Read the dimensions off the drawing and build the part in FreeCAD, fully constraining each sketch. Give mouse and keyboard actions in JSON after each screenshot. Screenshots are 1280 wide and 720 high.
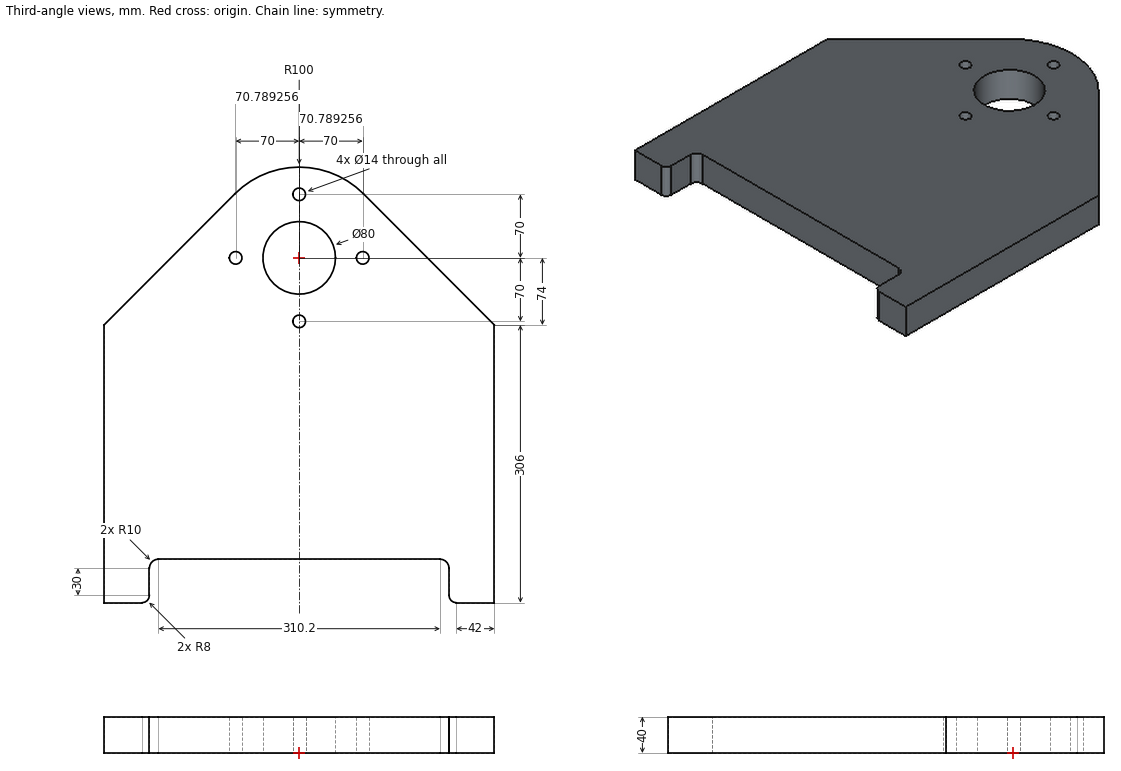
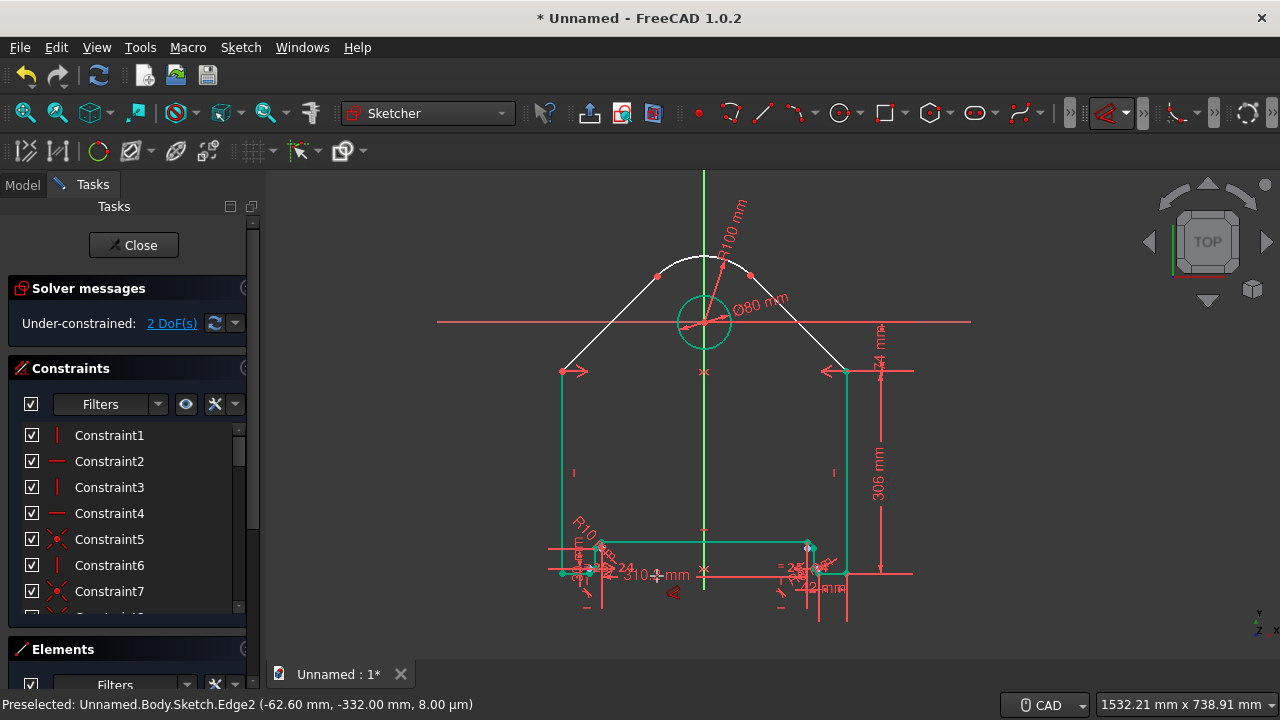
{"action": "left_click", "coordinate": [751, 275]}
{"action": "left_click", "coordinate": [728, 356]}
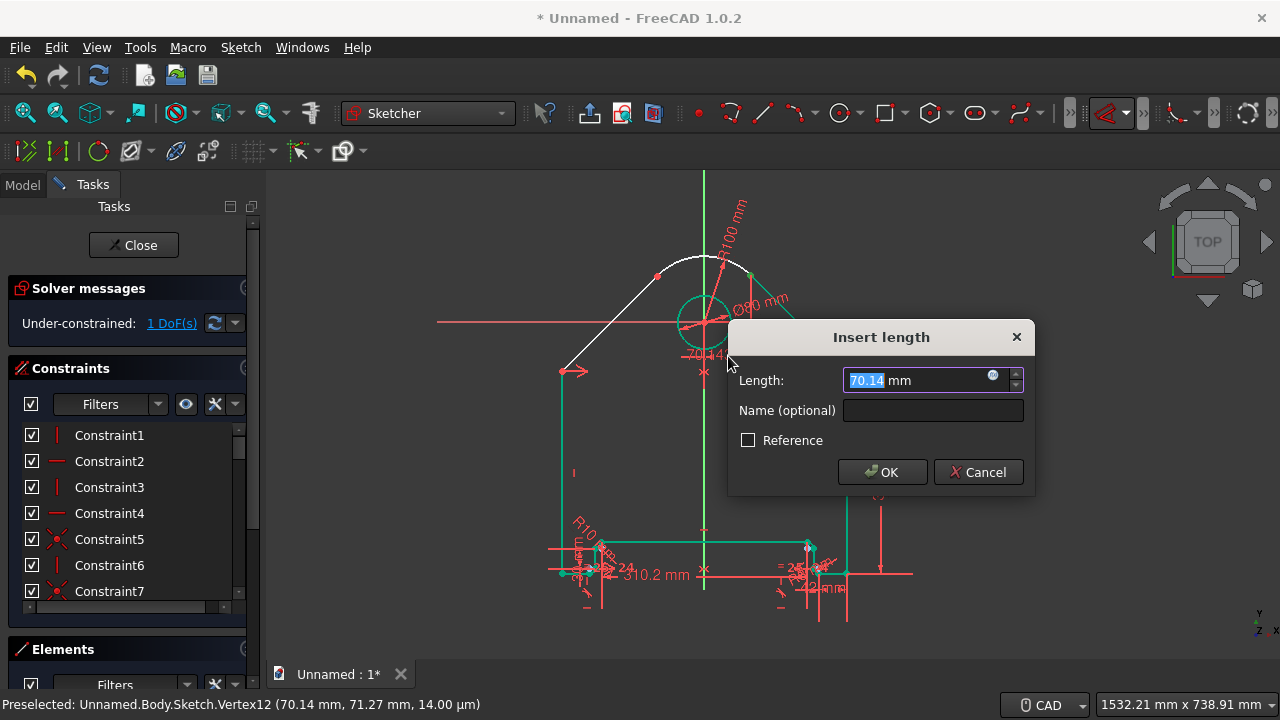
{"action": "type", "text": "70.789256"}
{"action": "key", "text": "Return"}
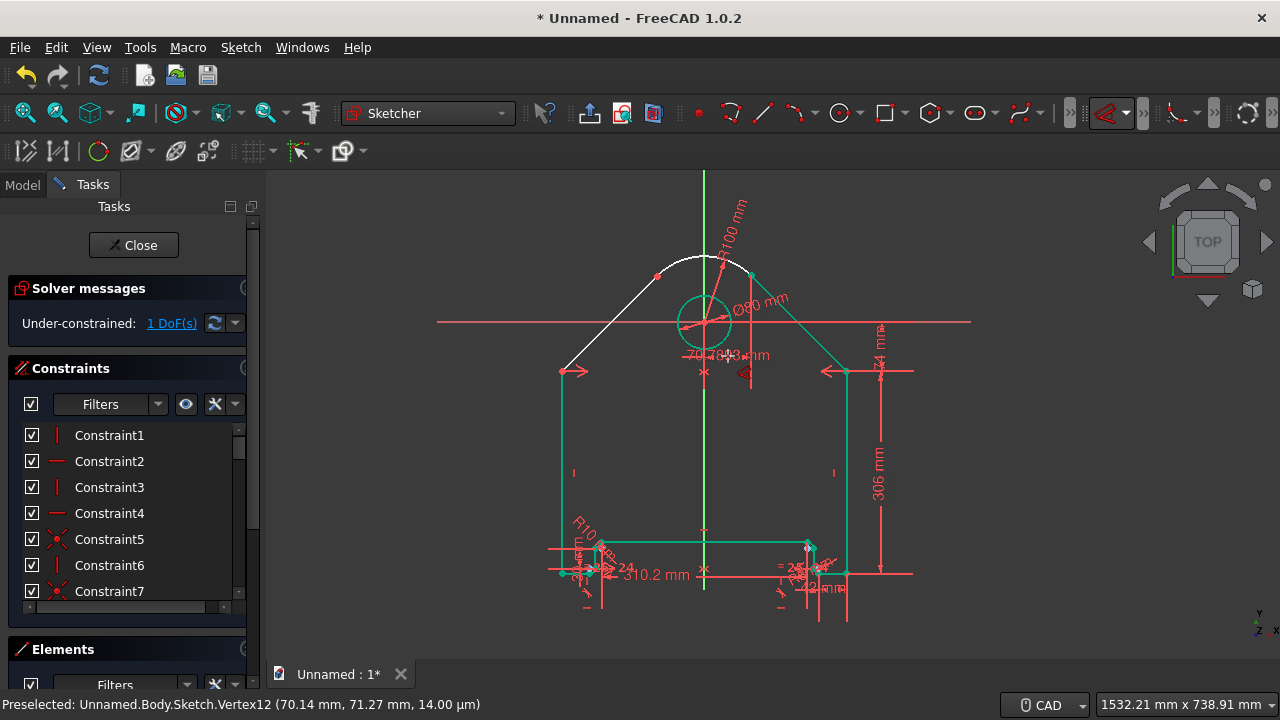
{"action": "left_click", "coordinate": [657, 276]}
{"action": "left_click", "coordinate": [664, 242]}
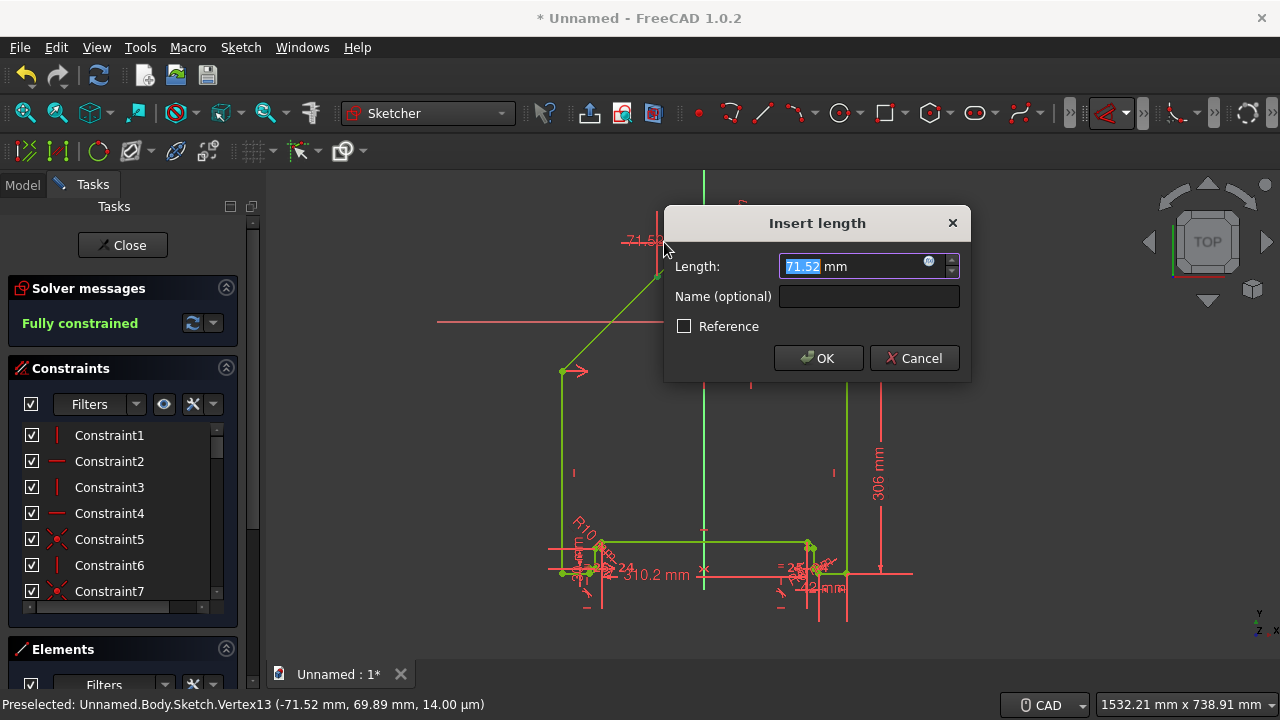
{"action": "type", "text": "70.789256"}
{"action": "key", "text": "Return"}
{"action": "key", "text": "Escape"}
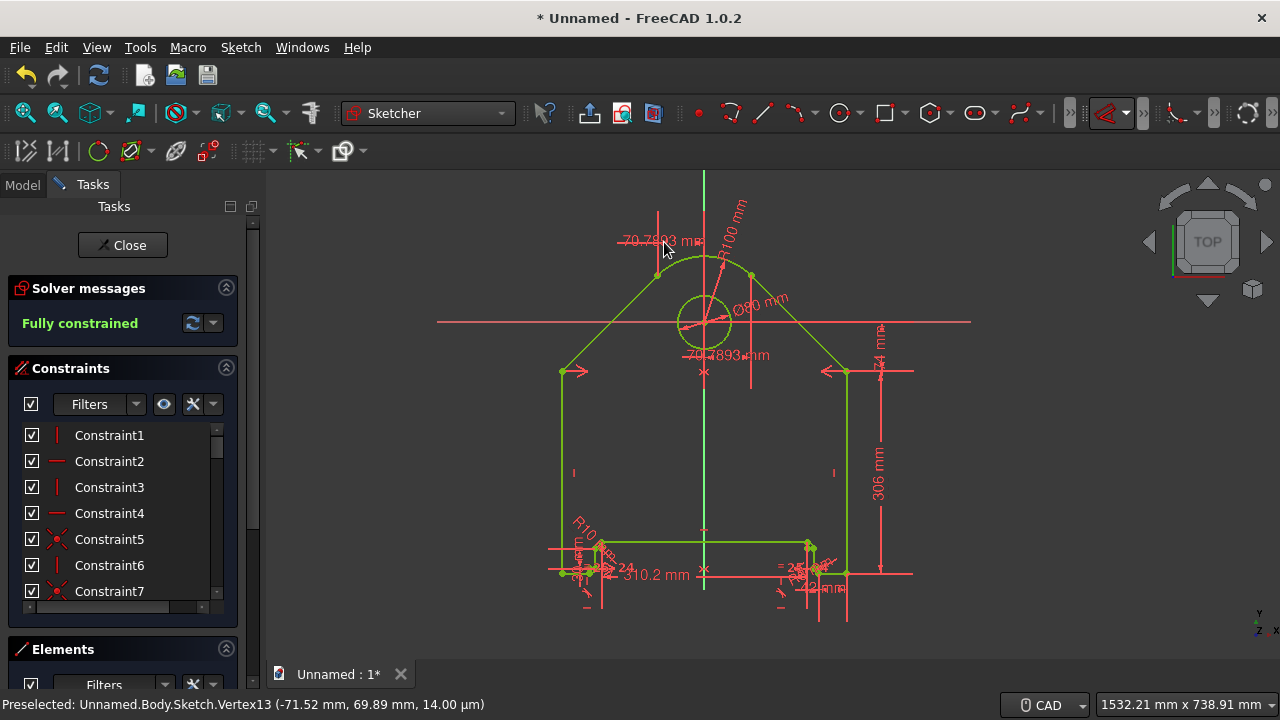
{"action": "left_click", "coordinate": [123, 245]}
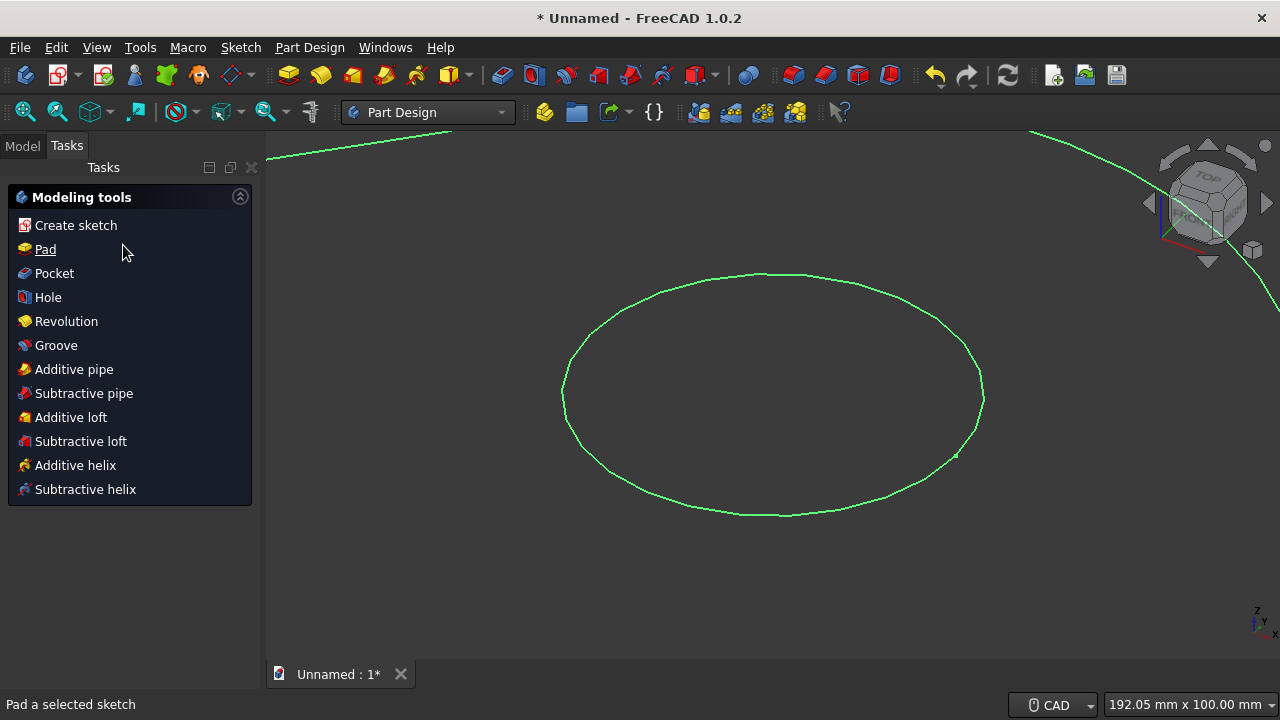
{"action": "left_click", "coordinate": [290, 76]}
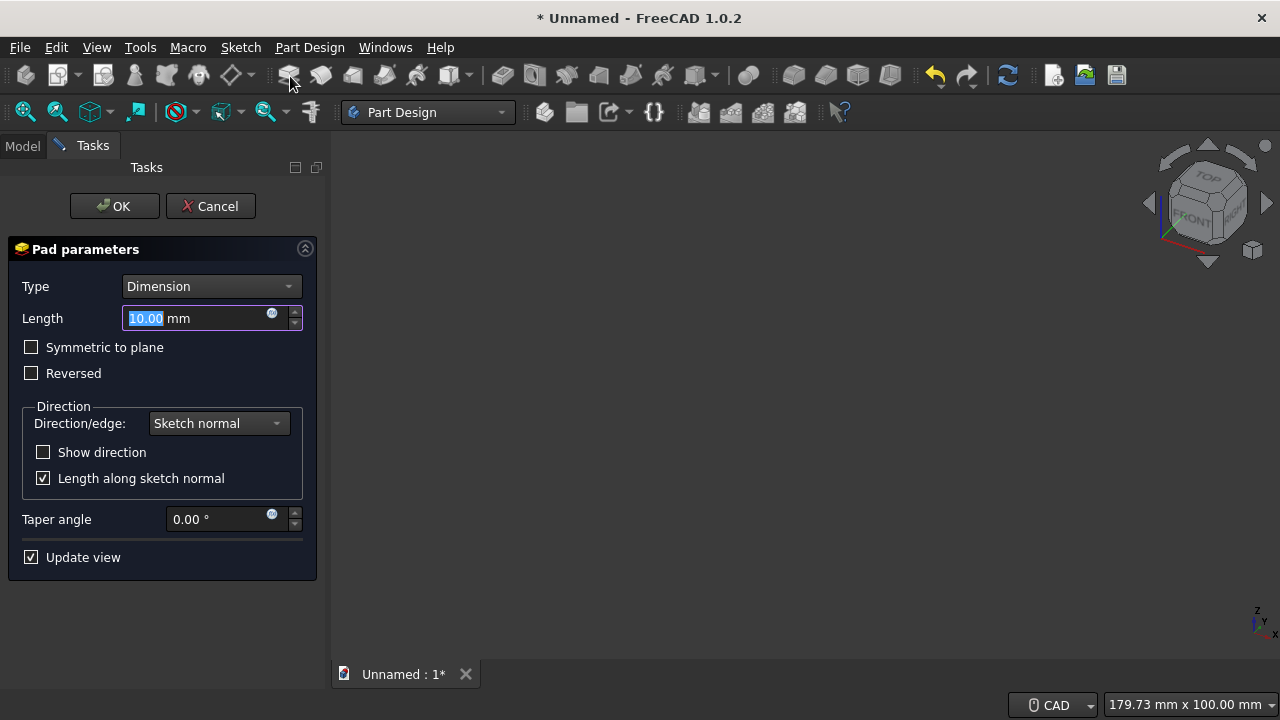
{"action": "type", "text": "40"}
{"action": "key", "text": "Tab"}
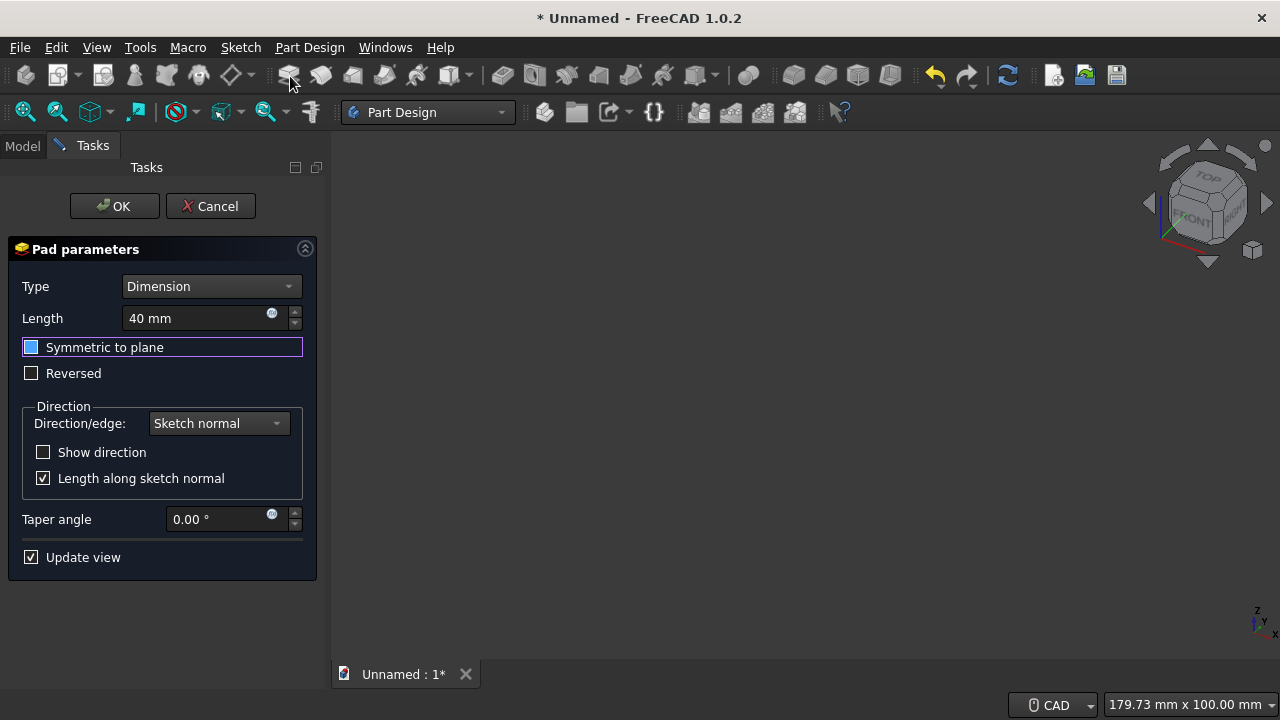
{"action": "left_click", "coordinate": [115, 206]}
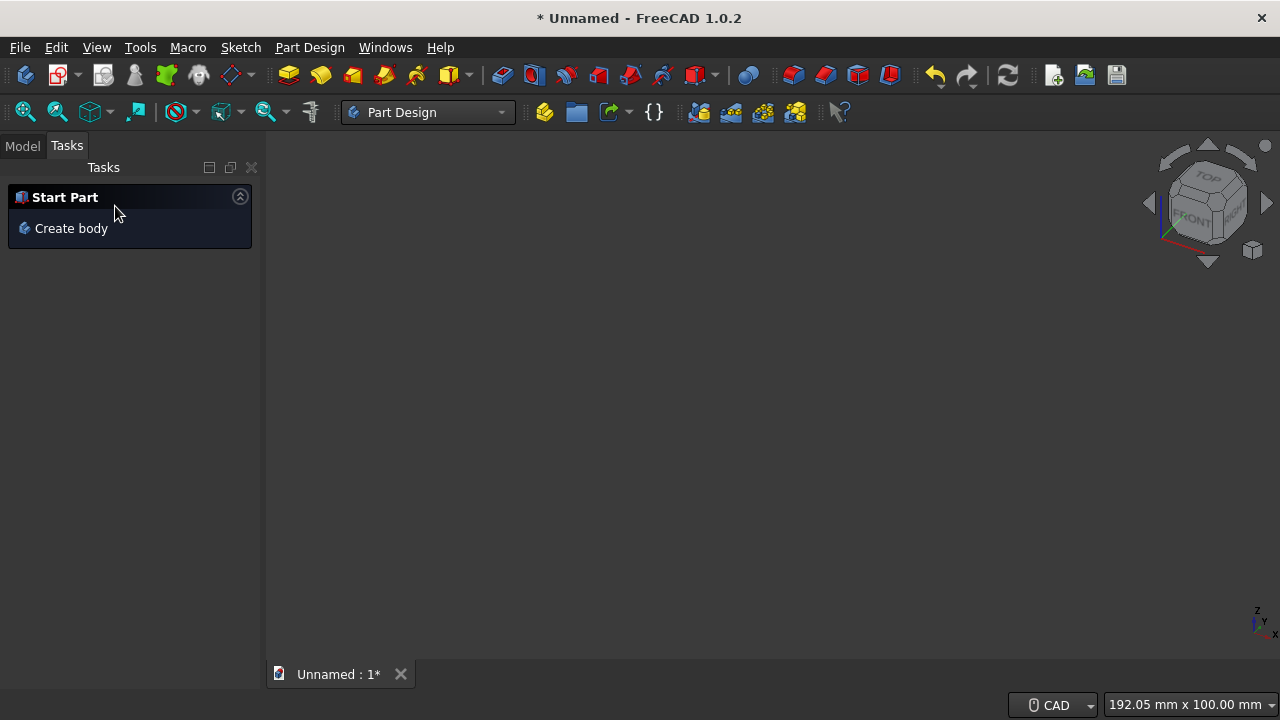
{"action": "key", "text": "v f"}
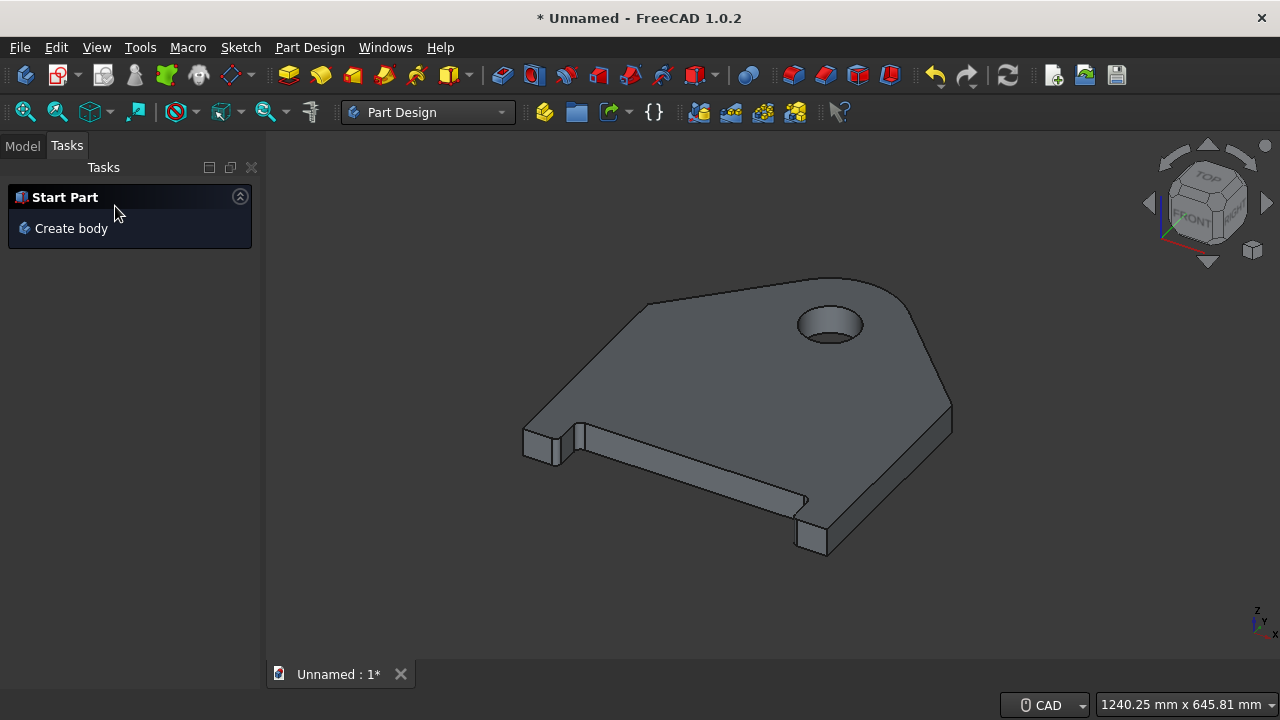
{"action": "left_click", "coordinate": [788, 423]}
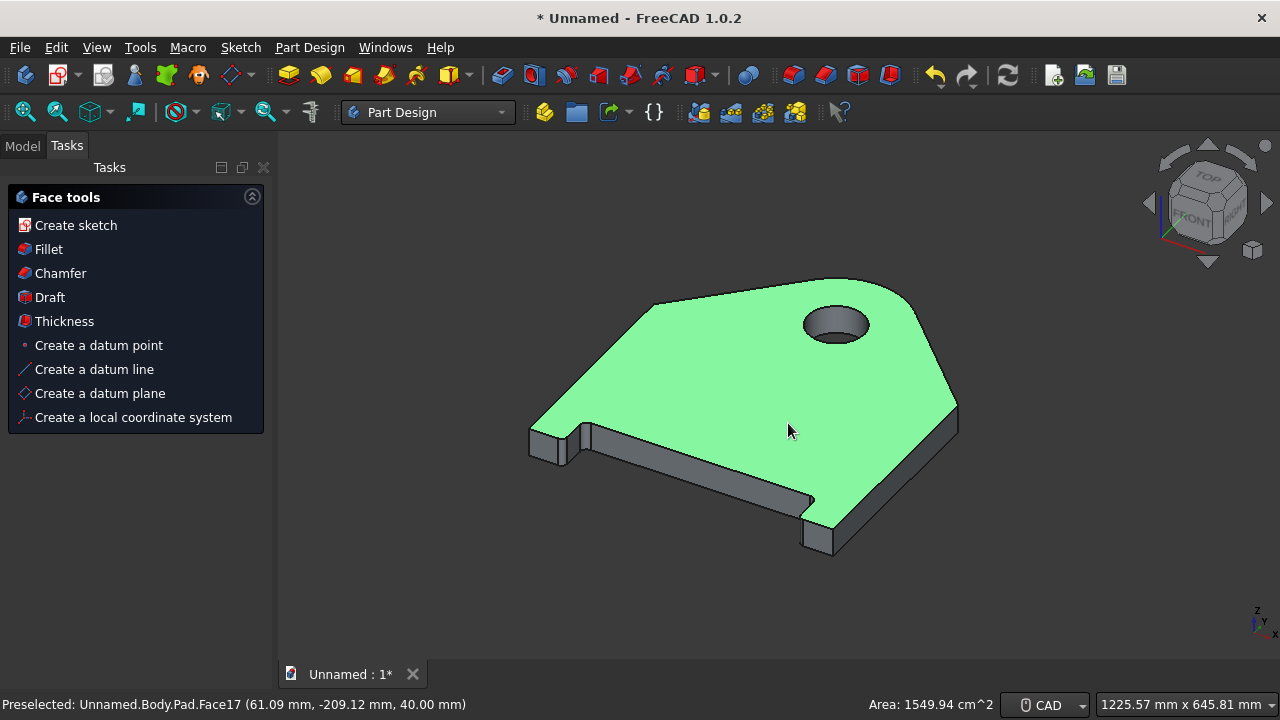
{"action": "left_click", "coordinate": [58, 76]}